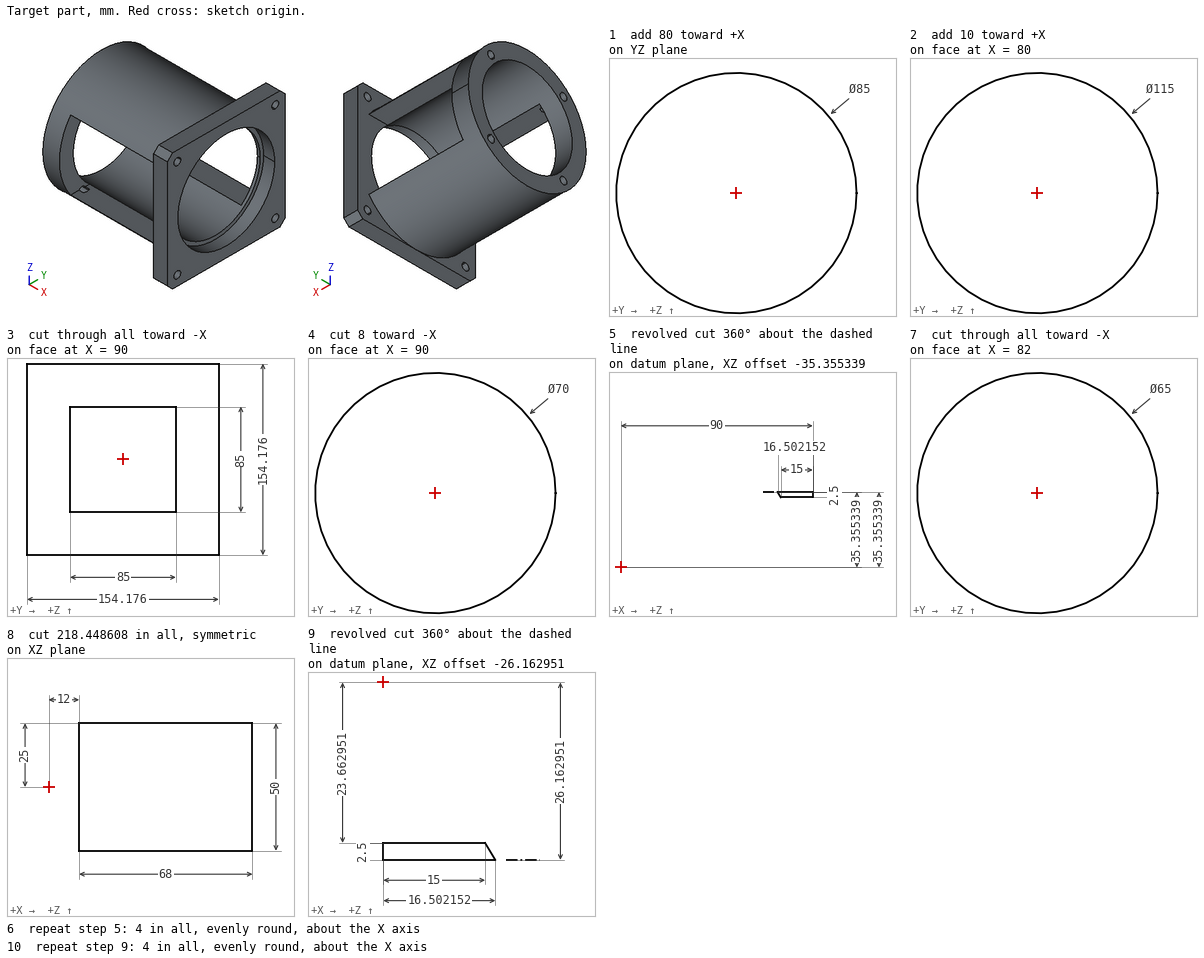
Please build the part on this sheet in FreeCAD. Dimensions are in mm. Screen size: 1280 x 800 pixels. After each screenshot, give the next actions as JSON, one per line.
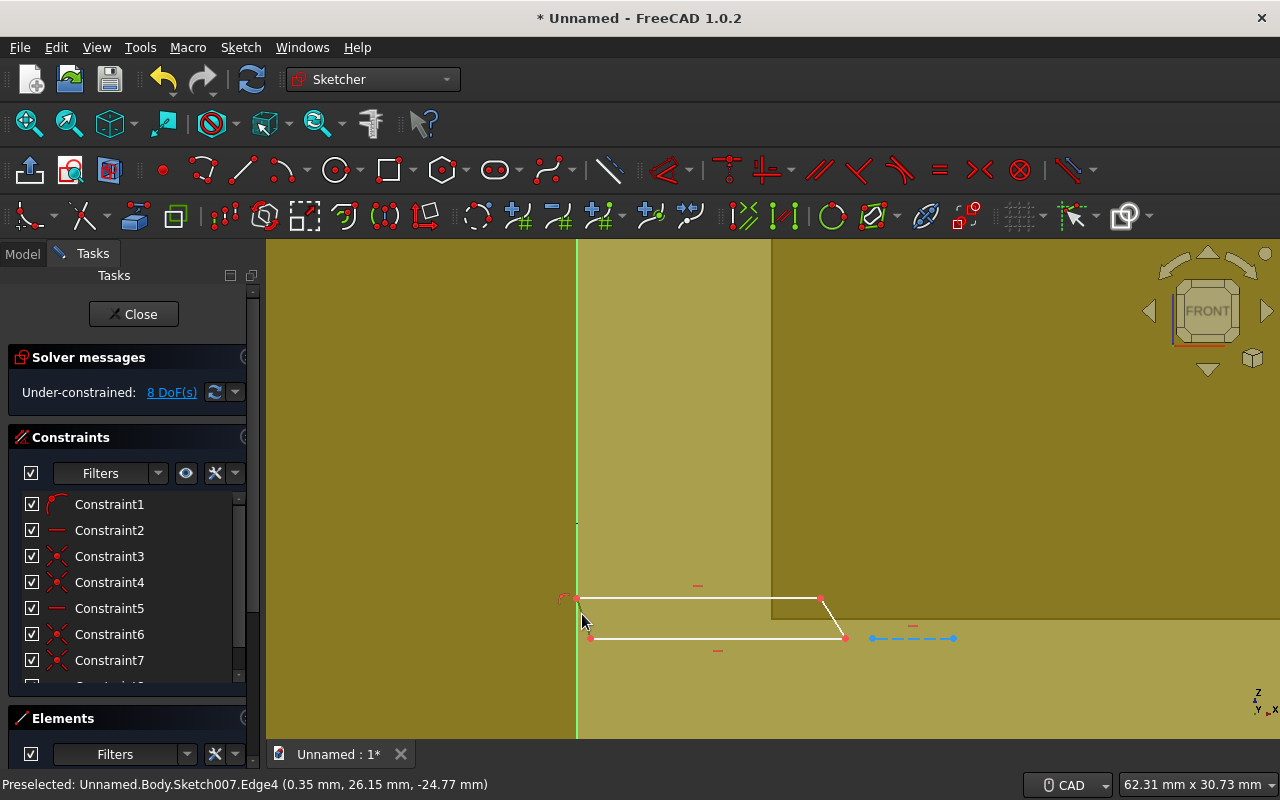
{"action": "key", "text": "v"}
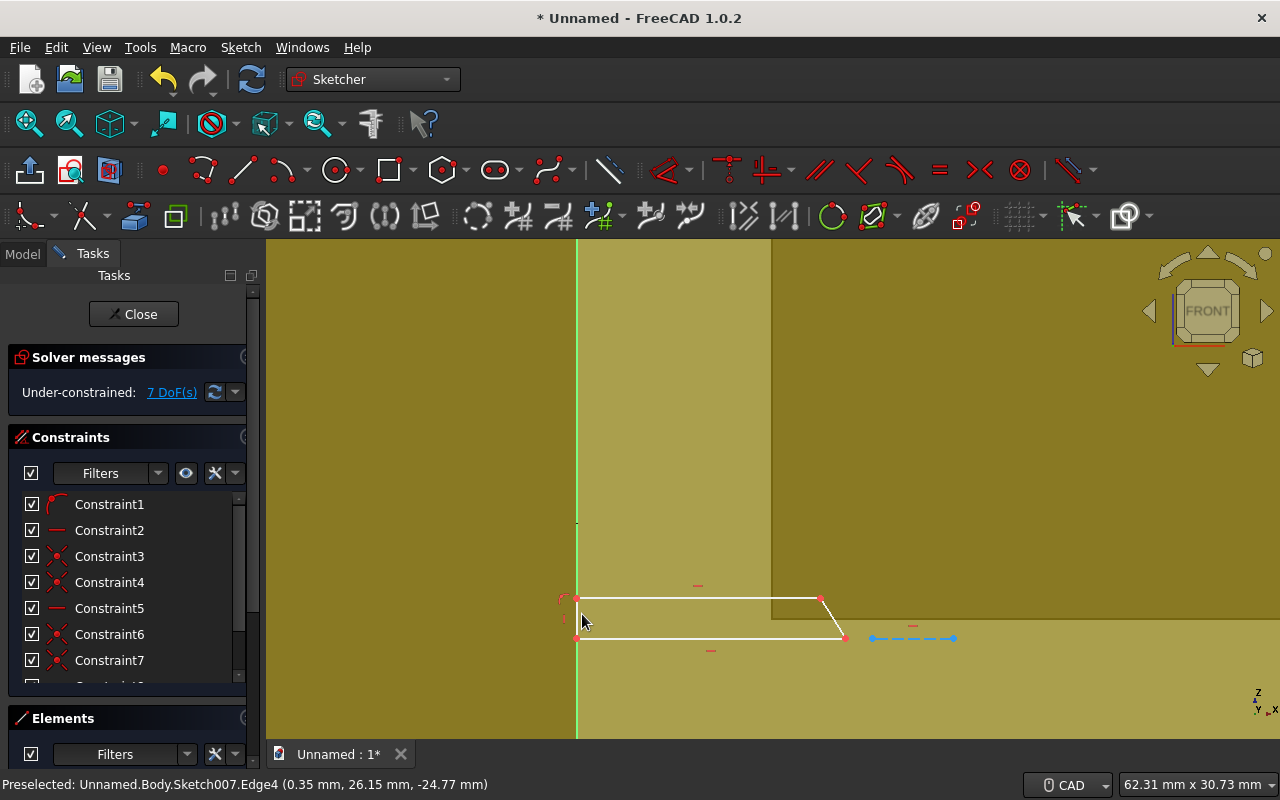
{"action": "left_click", "coordinate": [664, 170]}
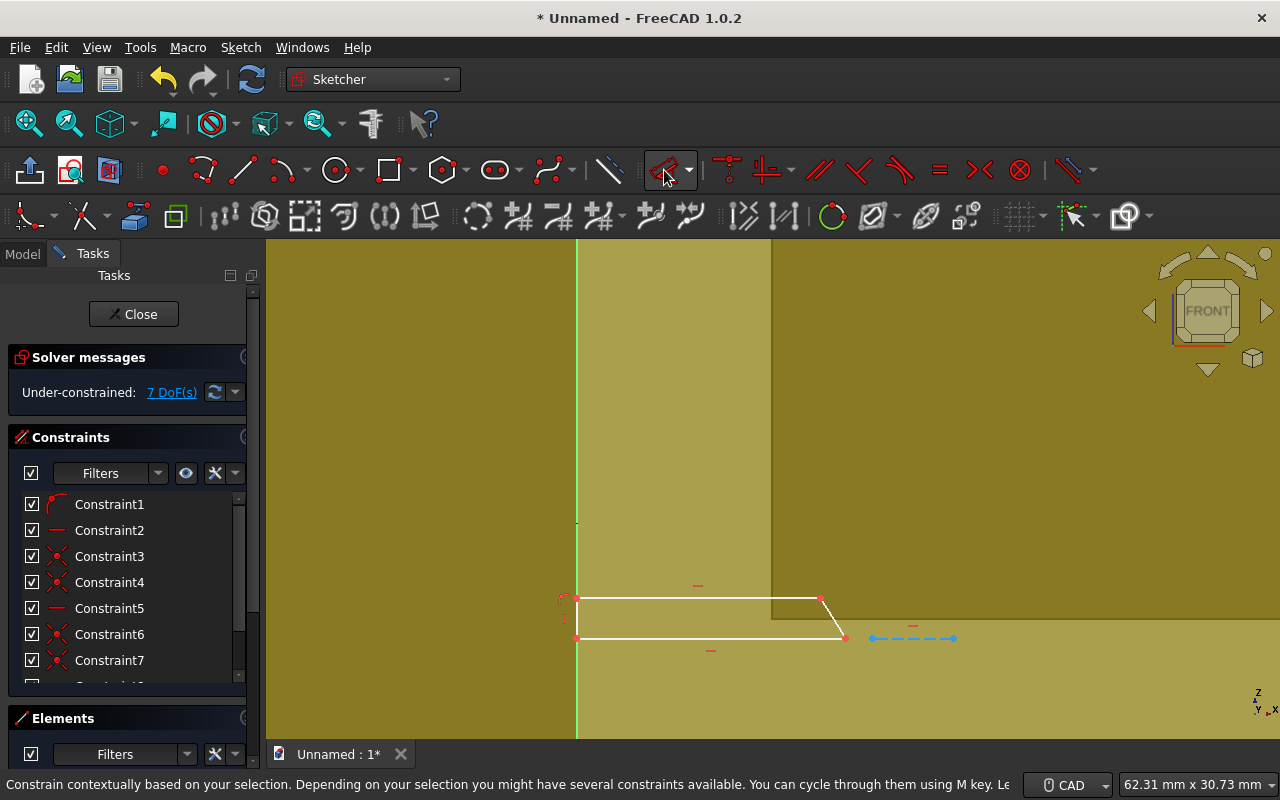
{"action": "left_click", "coordinate": [650, 598]}
{"action": "left_click", "coordinate": [699, 564]}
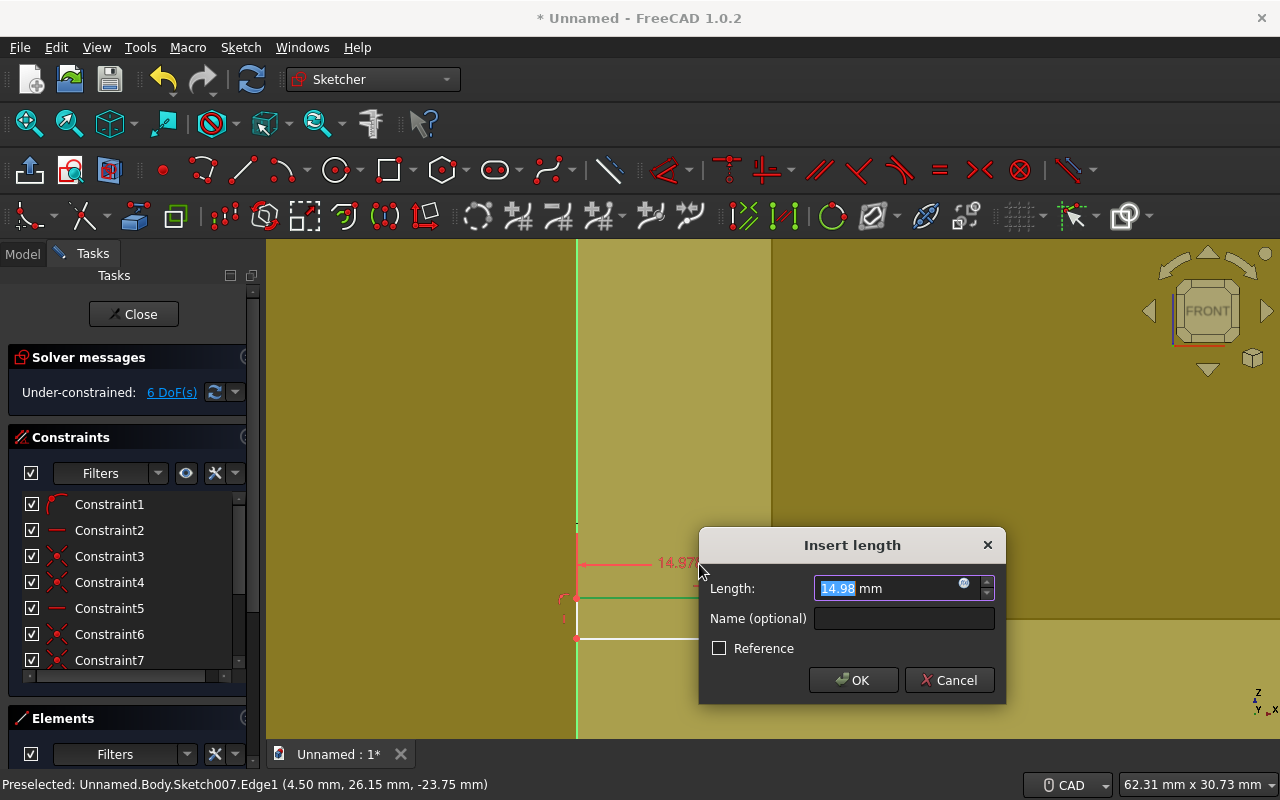
{"action": "type", "text": "15"}
{"action": "key", "text": "Return"}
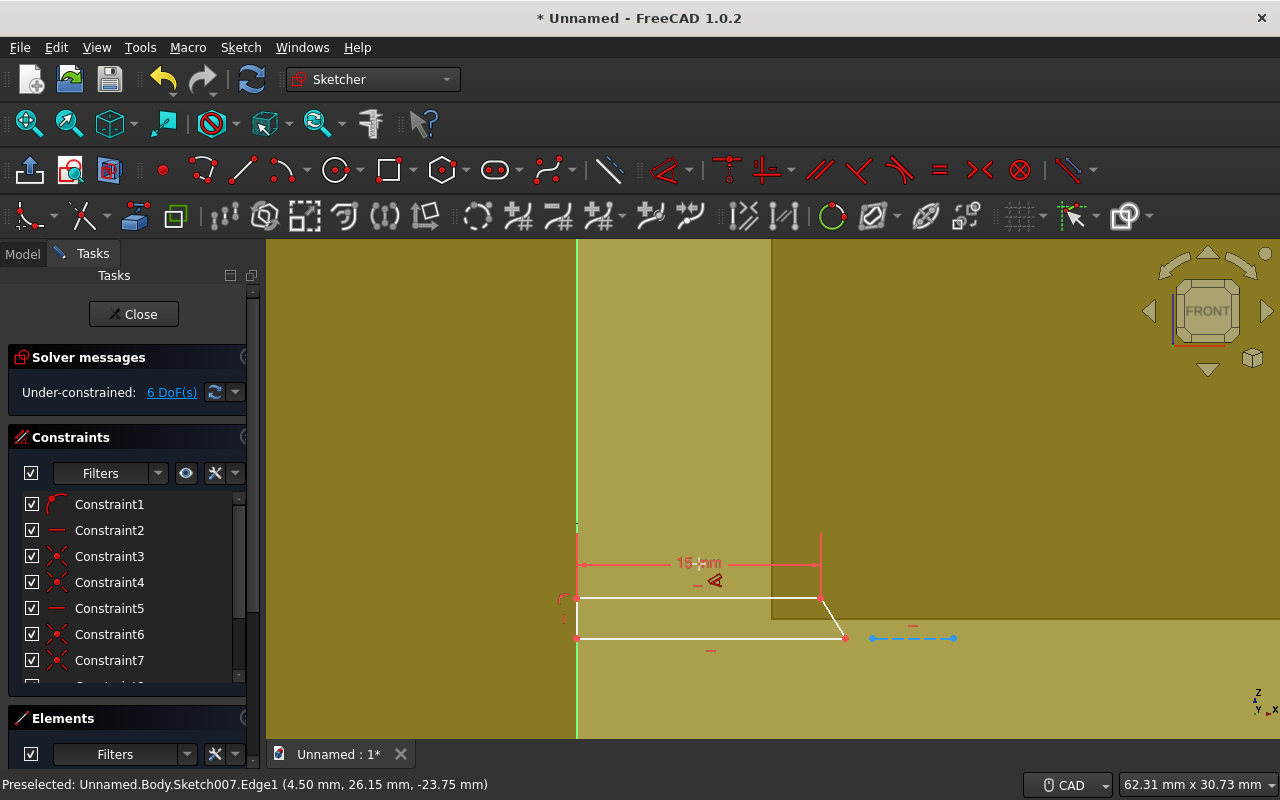
{"action": "left_click", "coordinate": [577, 626]}
{"action": "left_click", "coordinate": [543, 618]}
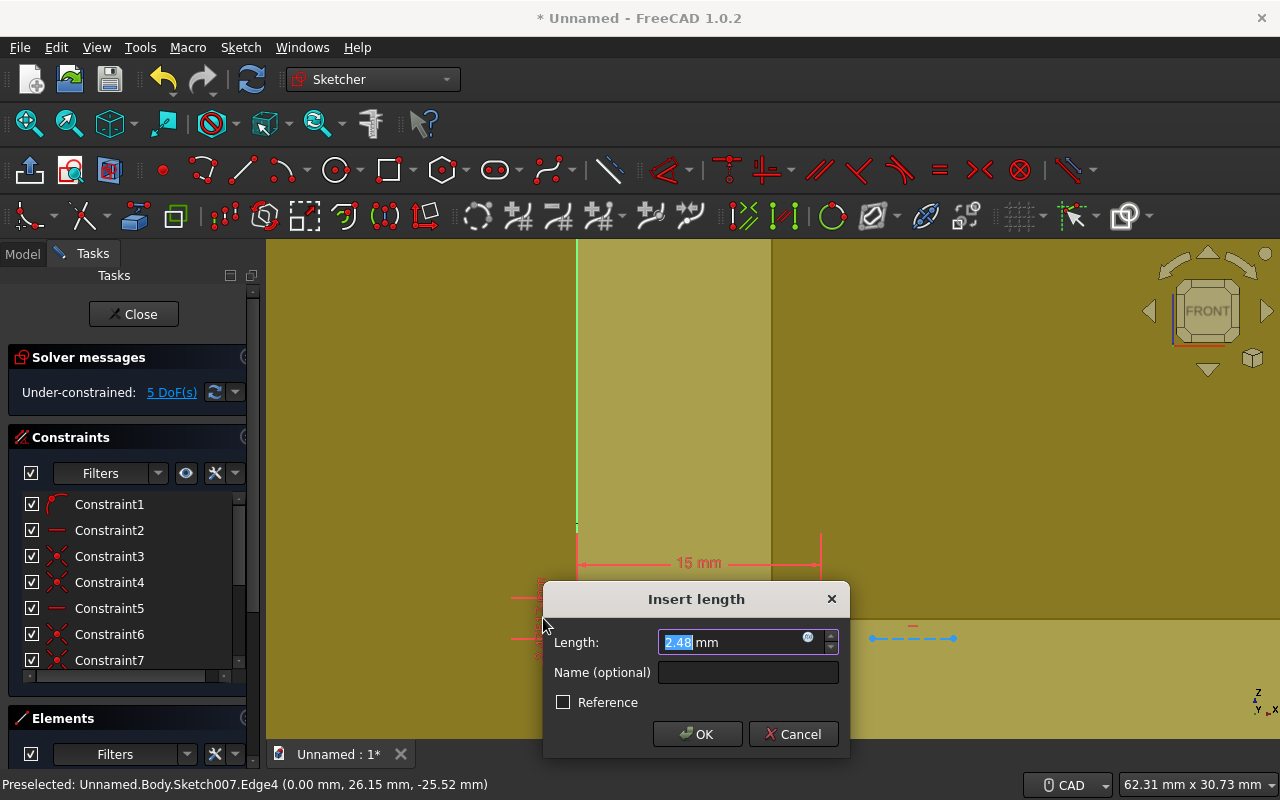
{"action": "type", "text": "2.5"}
{"action": "key", "text": "Return"}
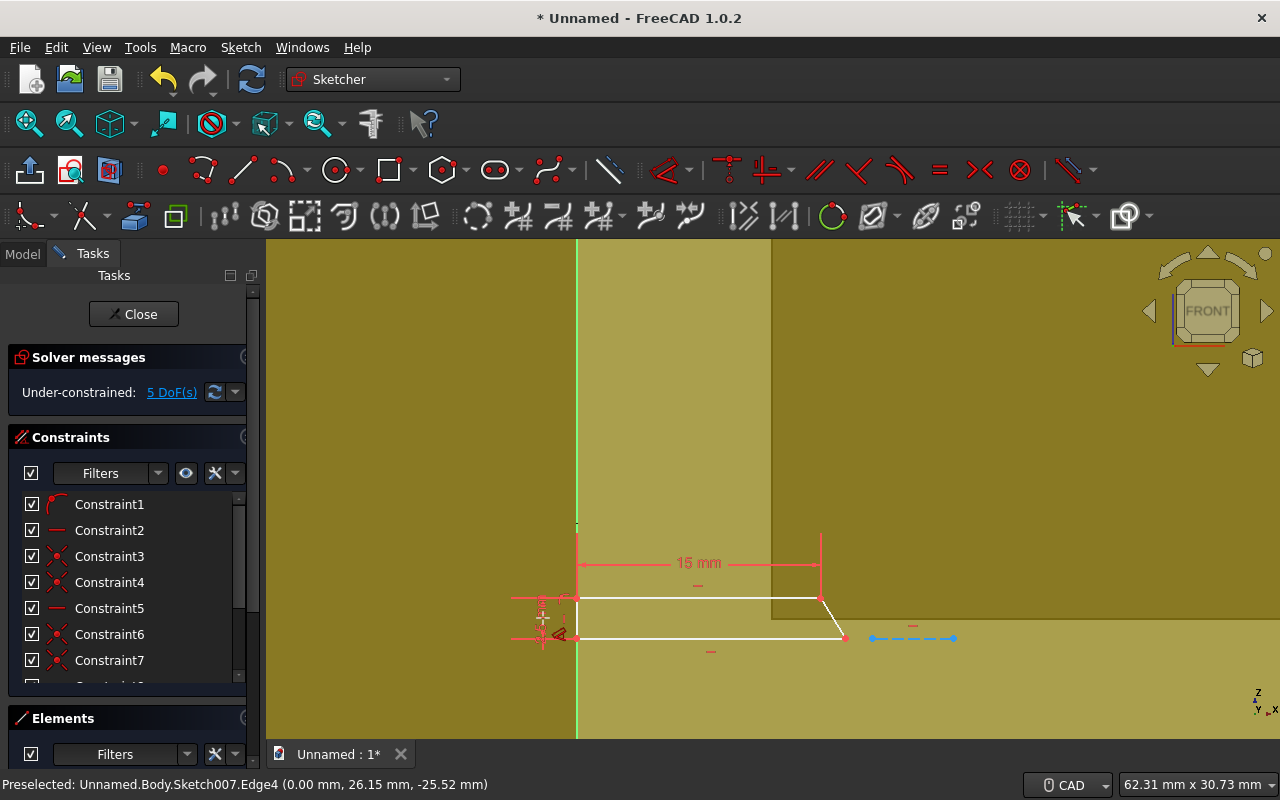
{"action": "left_click", "coordinate": [765, 639]}
{"action": "left_click", "coordinate": [711, 673]}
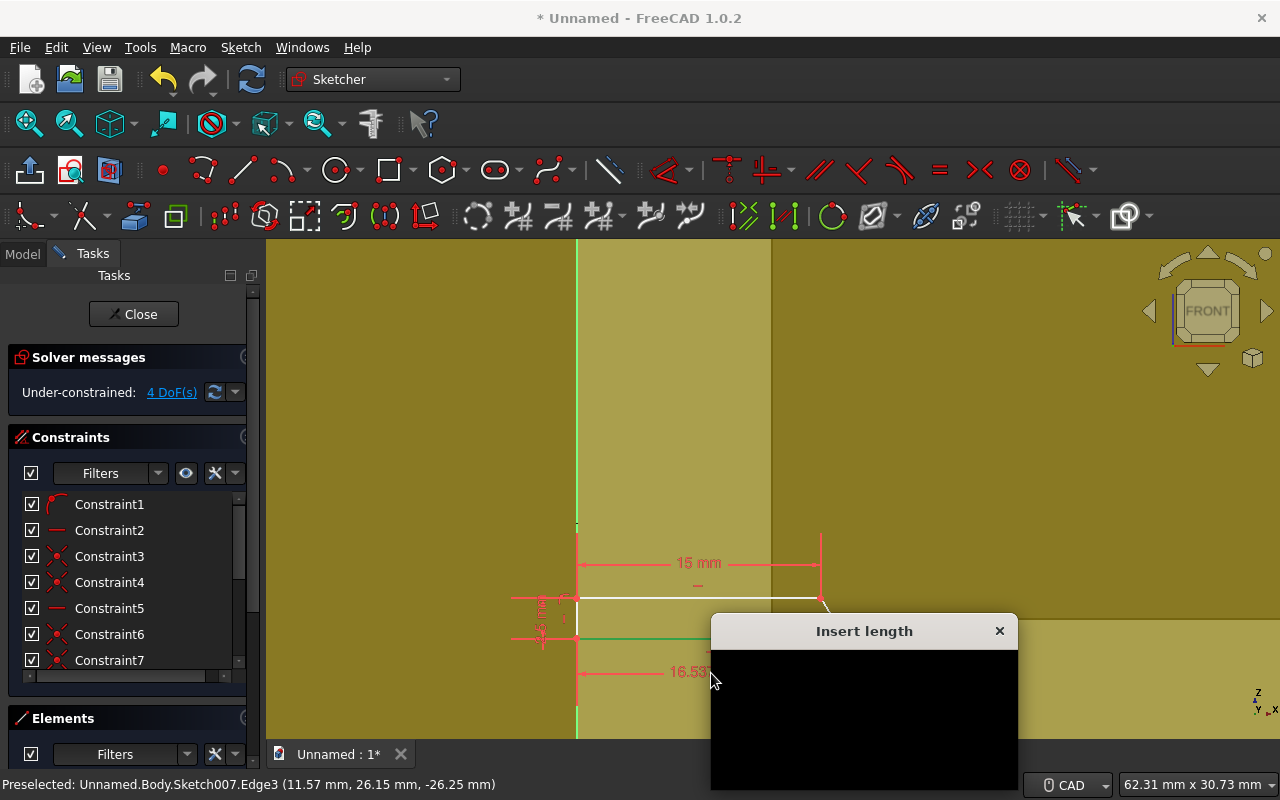
{"action": "type", "text": "16.502152"}
{"action": "key", "text": "Return"}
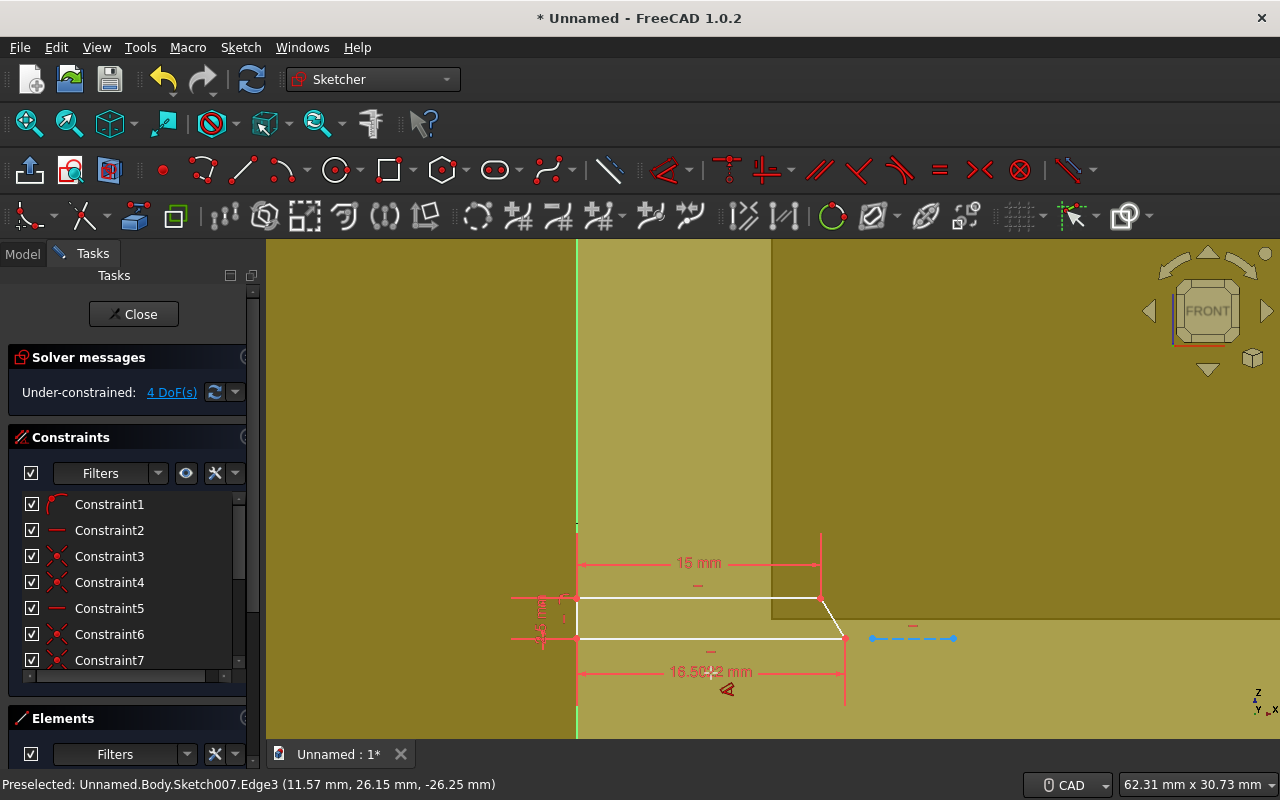
{"action": "left_click", "coordinate": [577, 598]}
{"action": "left_click", "coordinate": [543, 433]}